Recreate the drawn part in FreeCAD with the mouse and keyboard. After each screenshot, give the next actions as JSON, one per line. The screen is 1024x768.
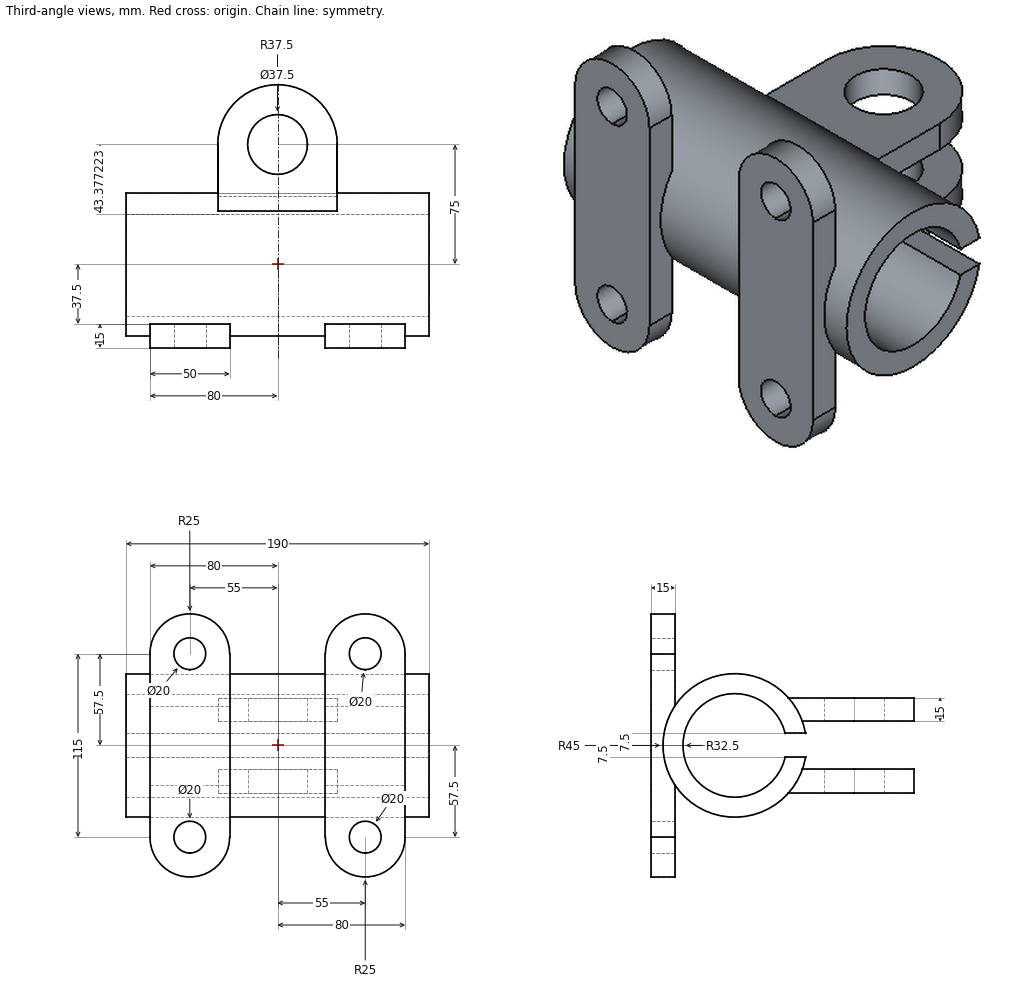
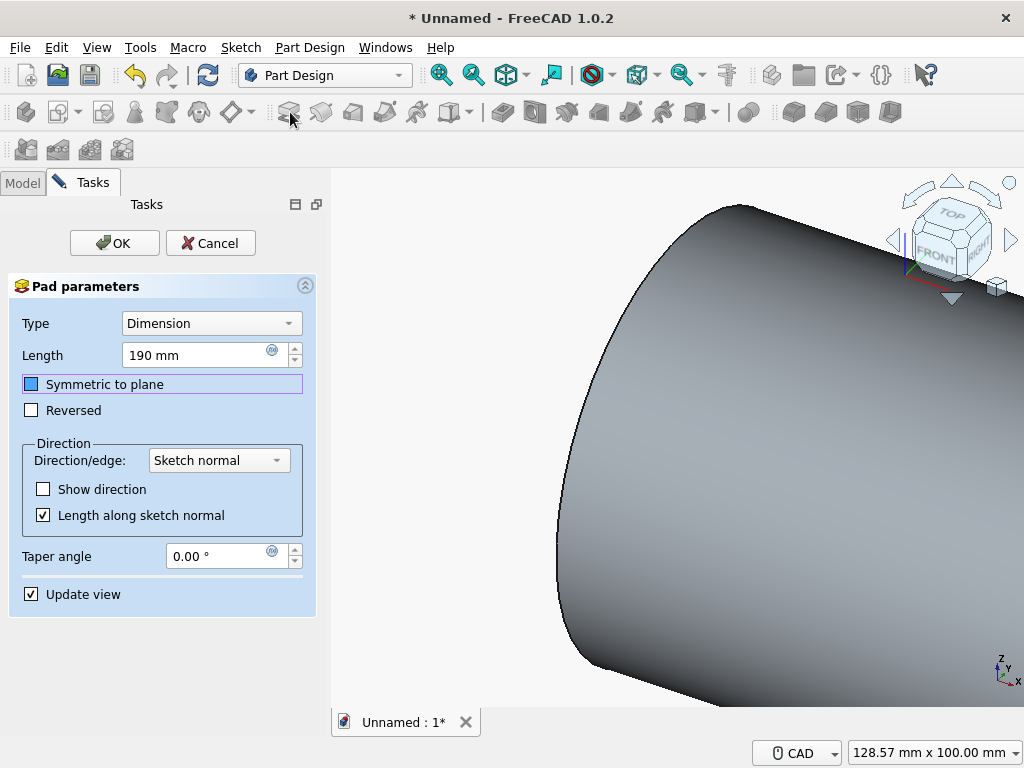
{"action": "left_click", "coordinate": [30, 384]}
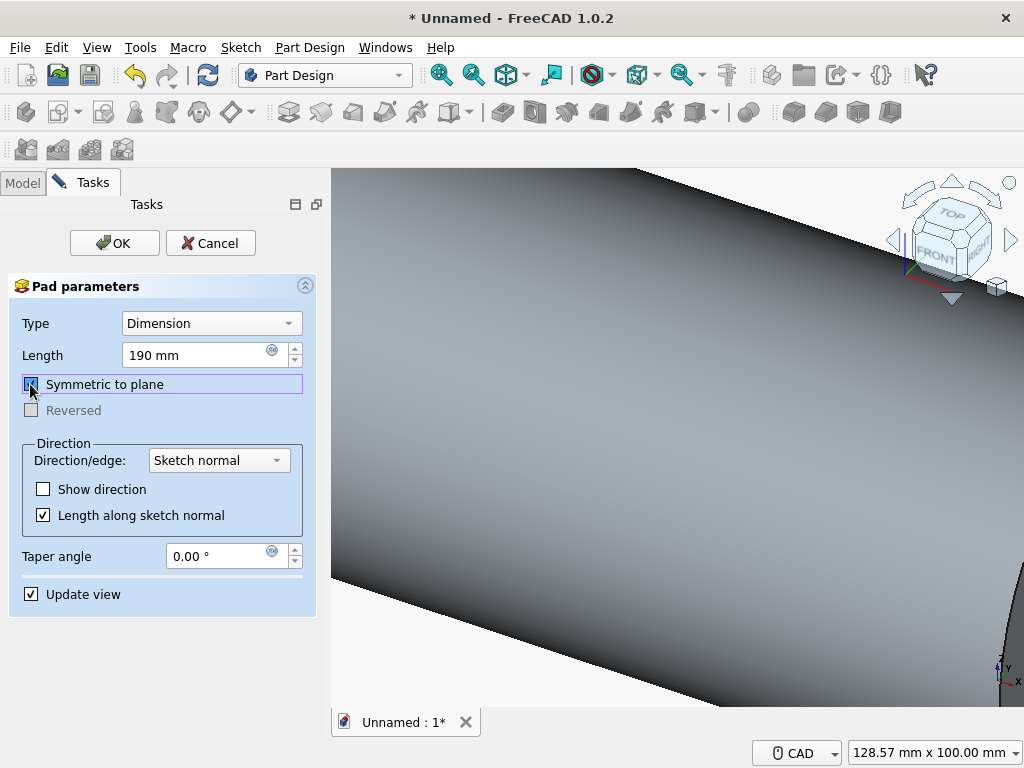
{"action": "left_click", "coordinate": [115, 243]}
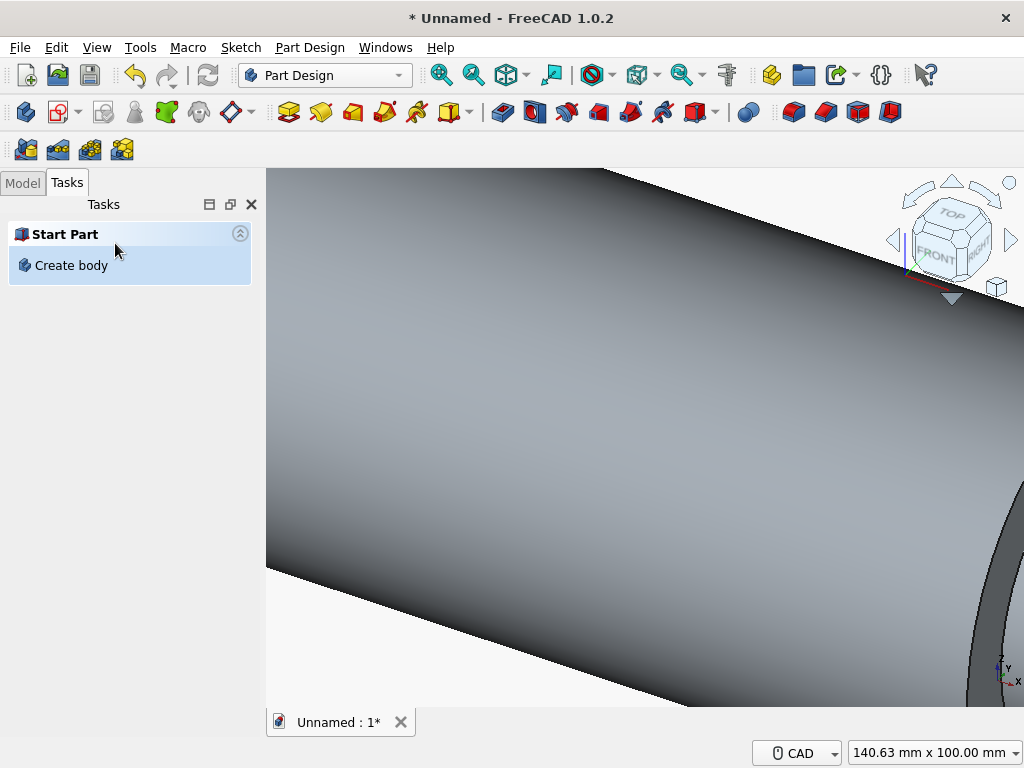
{"action": "left_click", "coordinate": [442, 76]}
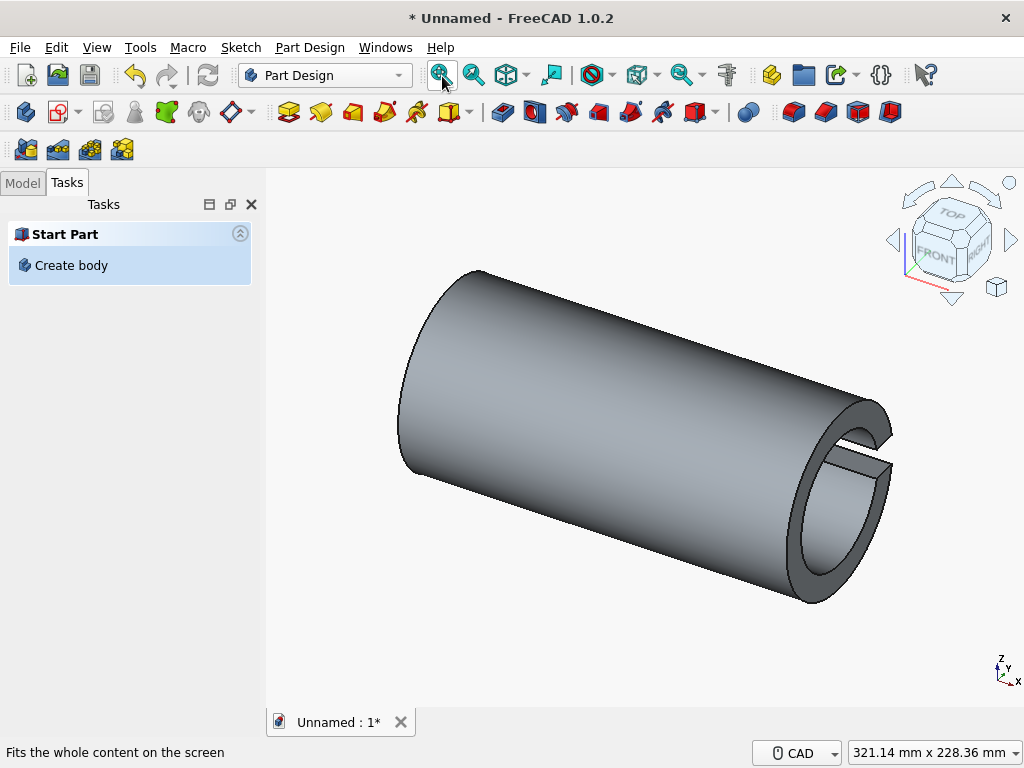
{"action": "left_click", "coordinate": [58, 112]}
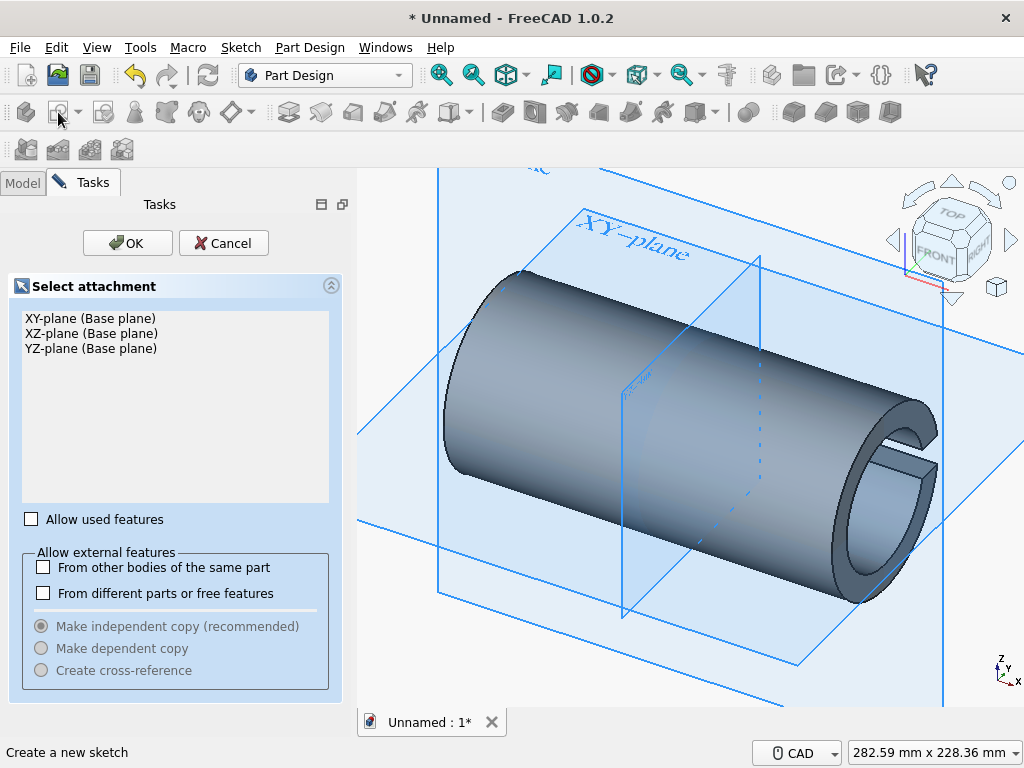
{"action": "left_click", "coordinate": [82, 318]}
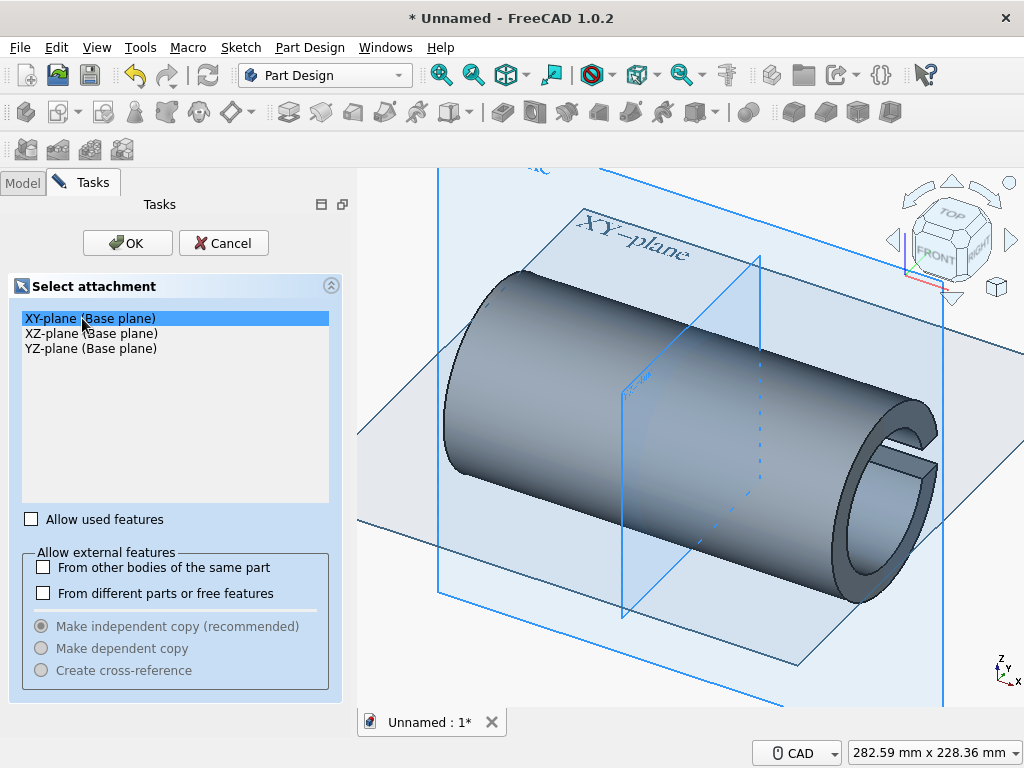
{"action": "left_click", "coordinate": [128, 243]}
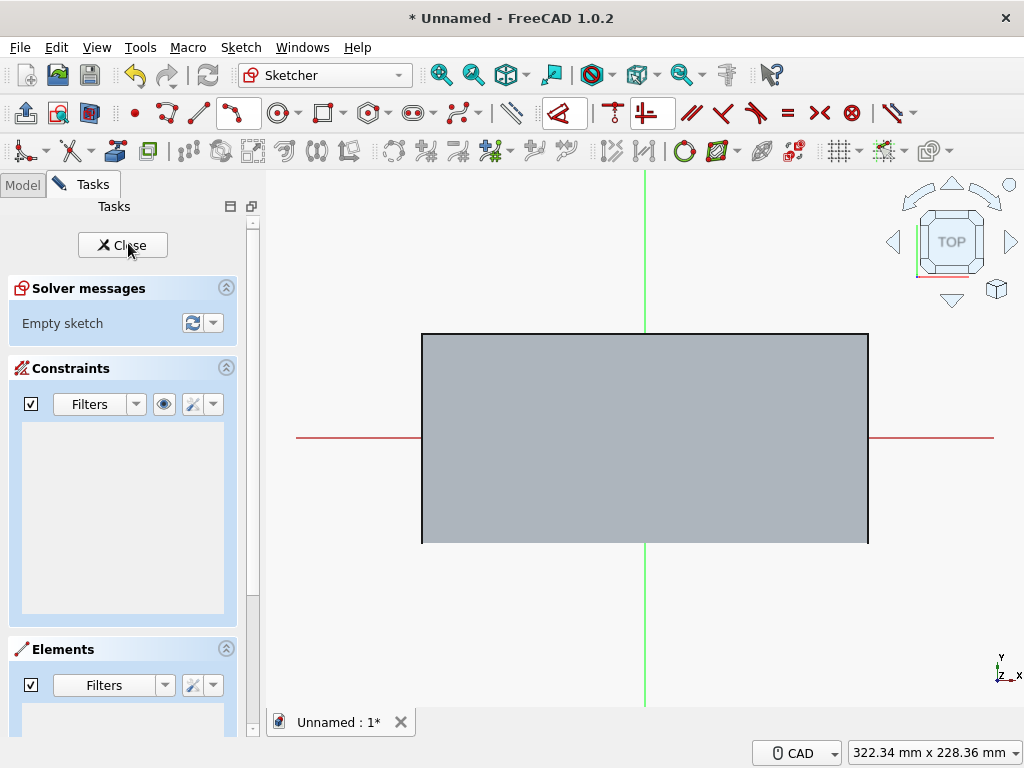
{"action": "left_click", "coordinate": [90, 114]}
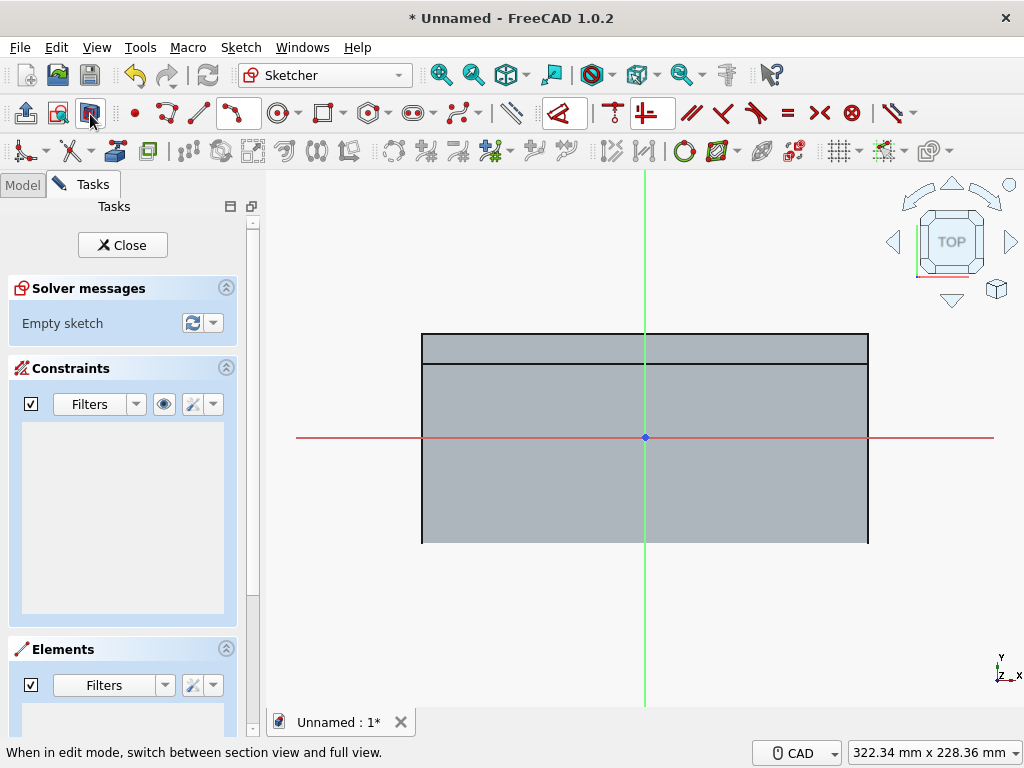
{"action": "left_click", "coordinate": [324, 114]}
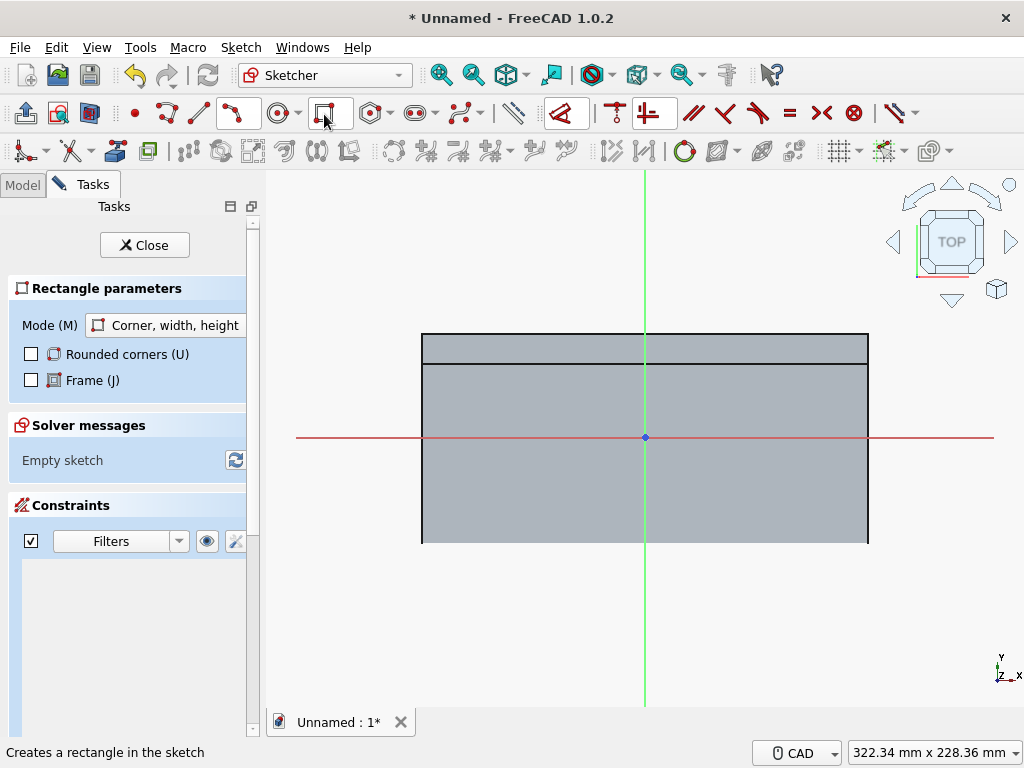
{"action": "left_click", "coordinate": [457, 526]}
{"action": "left_click", "coordinate": [574, 561]}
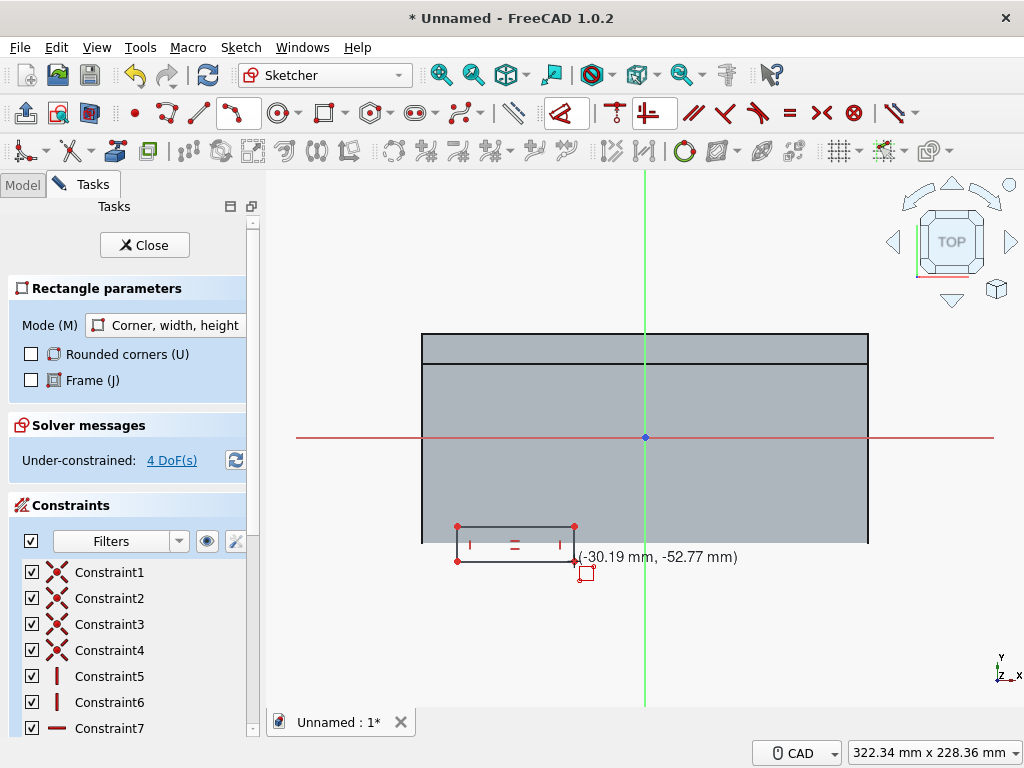
{"action": "left_click", "coordinate": [716, 526]}
{"action": "left_click", "coordinate": [833, 561]}
{"action": "key", "text": "Escape"}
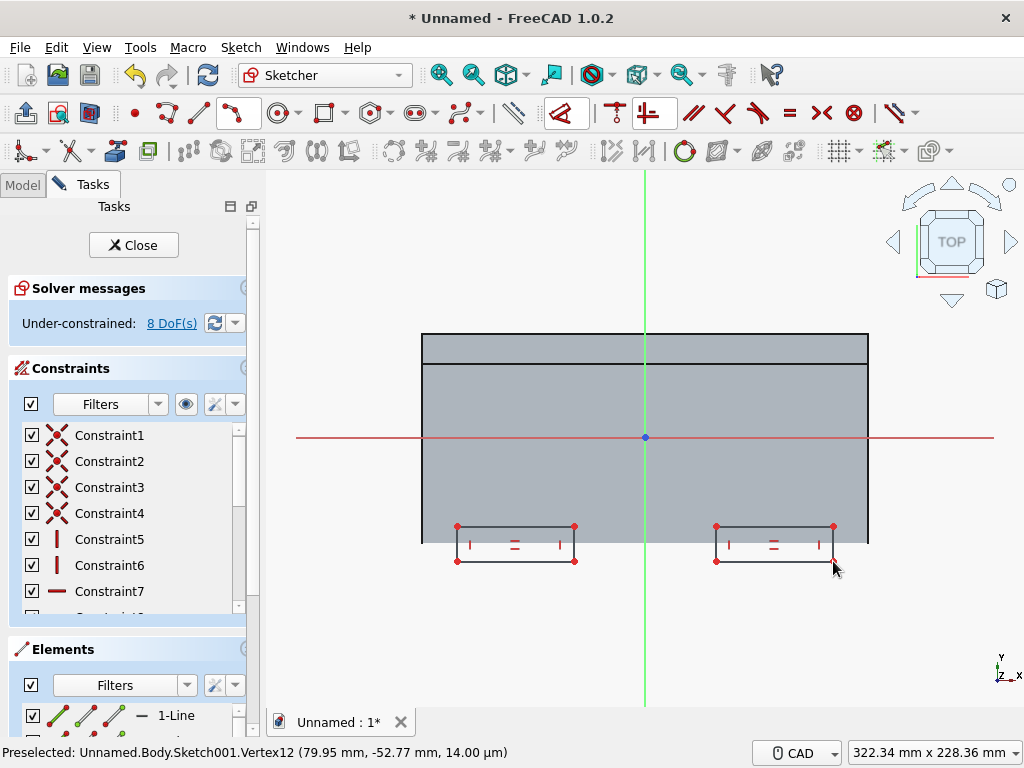
{"action": "left_click", "coordinate": [574, 527]}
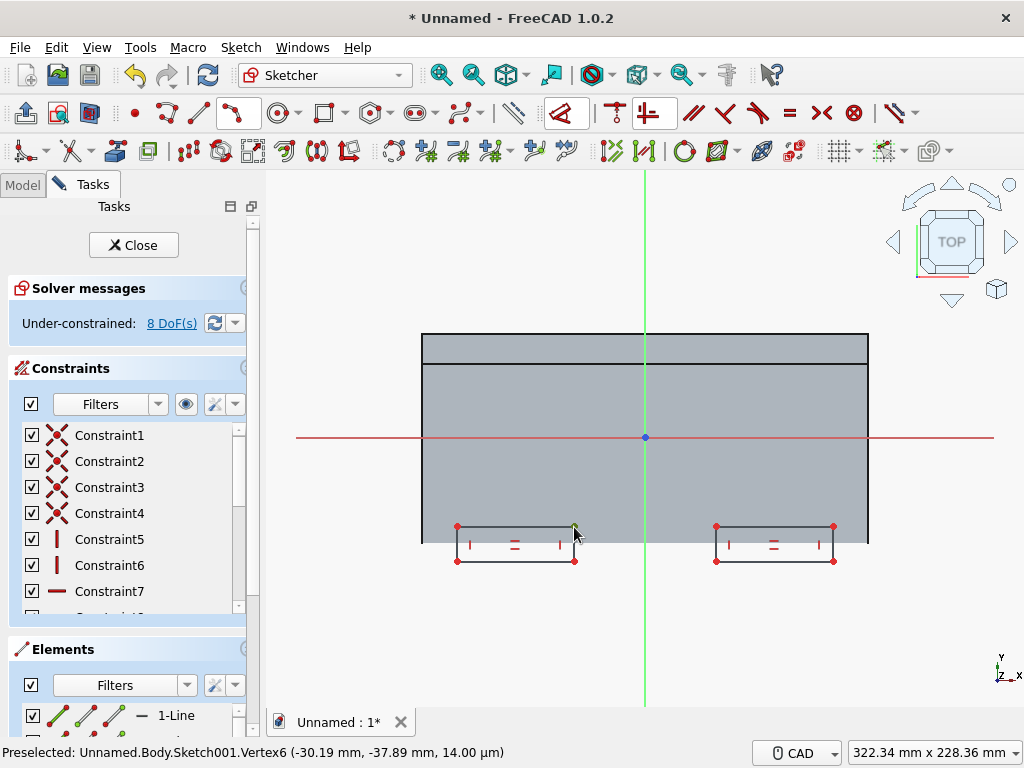
{"action": "left_click", "coordinate": [716, 527]}